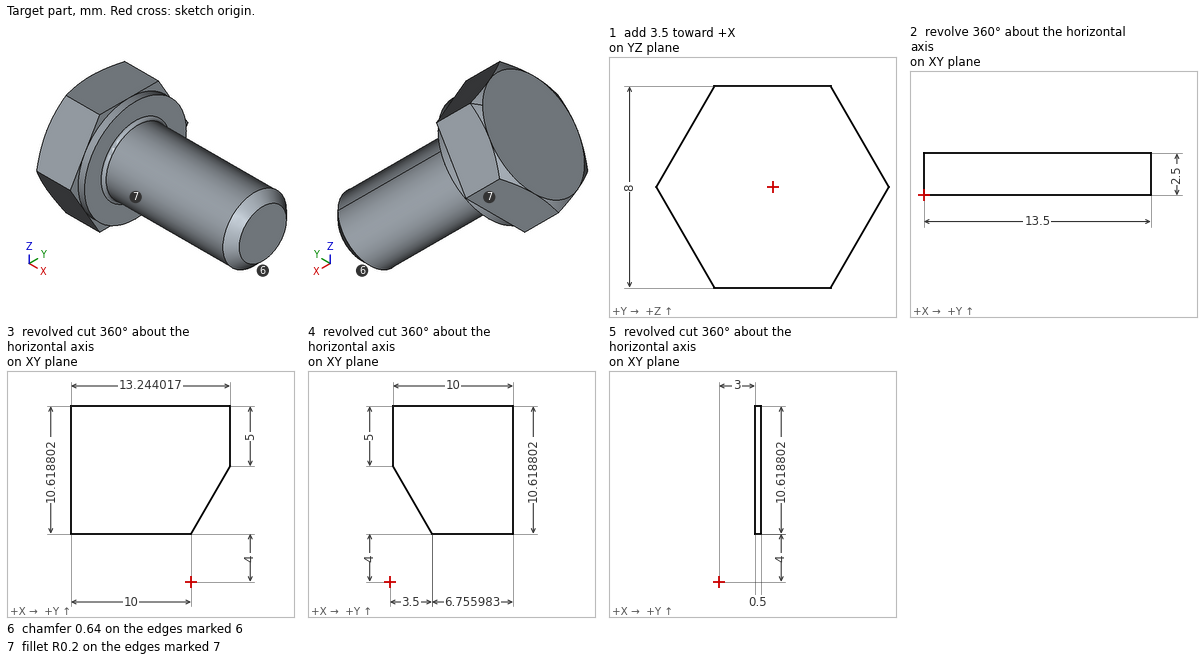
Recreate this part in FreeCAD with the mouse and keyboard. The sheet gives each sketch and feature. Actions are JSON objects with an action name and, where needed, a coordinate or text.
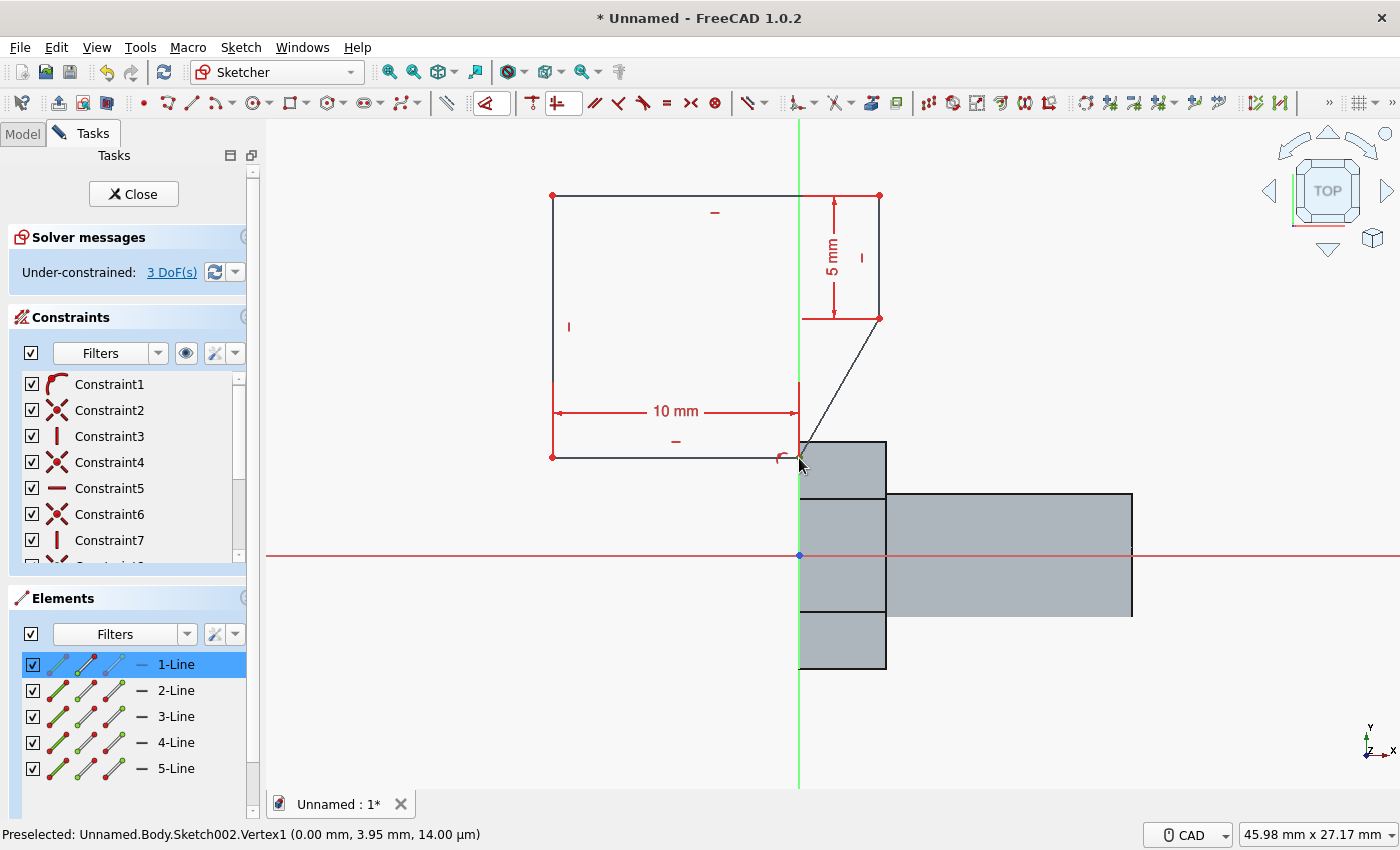
{"action": "key", "text": "i"}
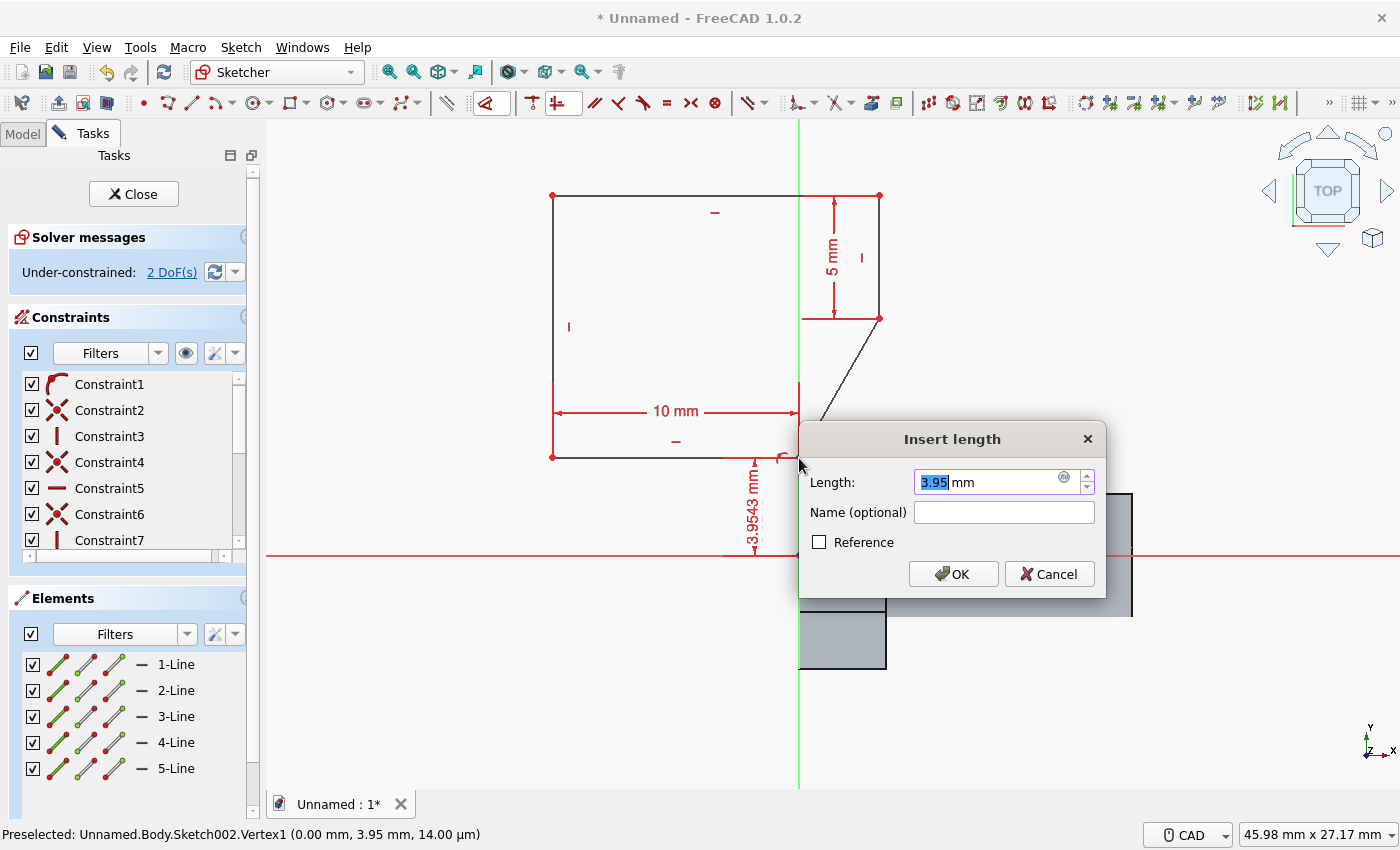
{"action": "type", "text": "4"}
{"action": "key", "text": "Return"}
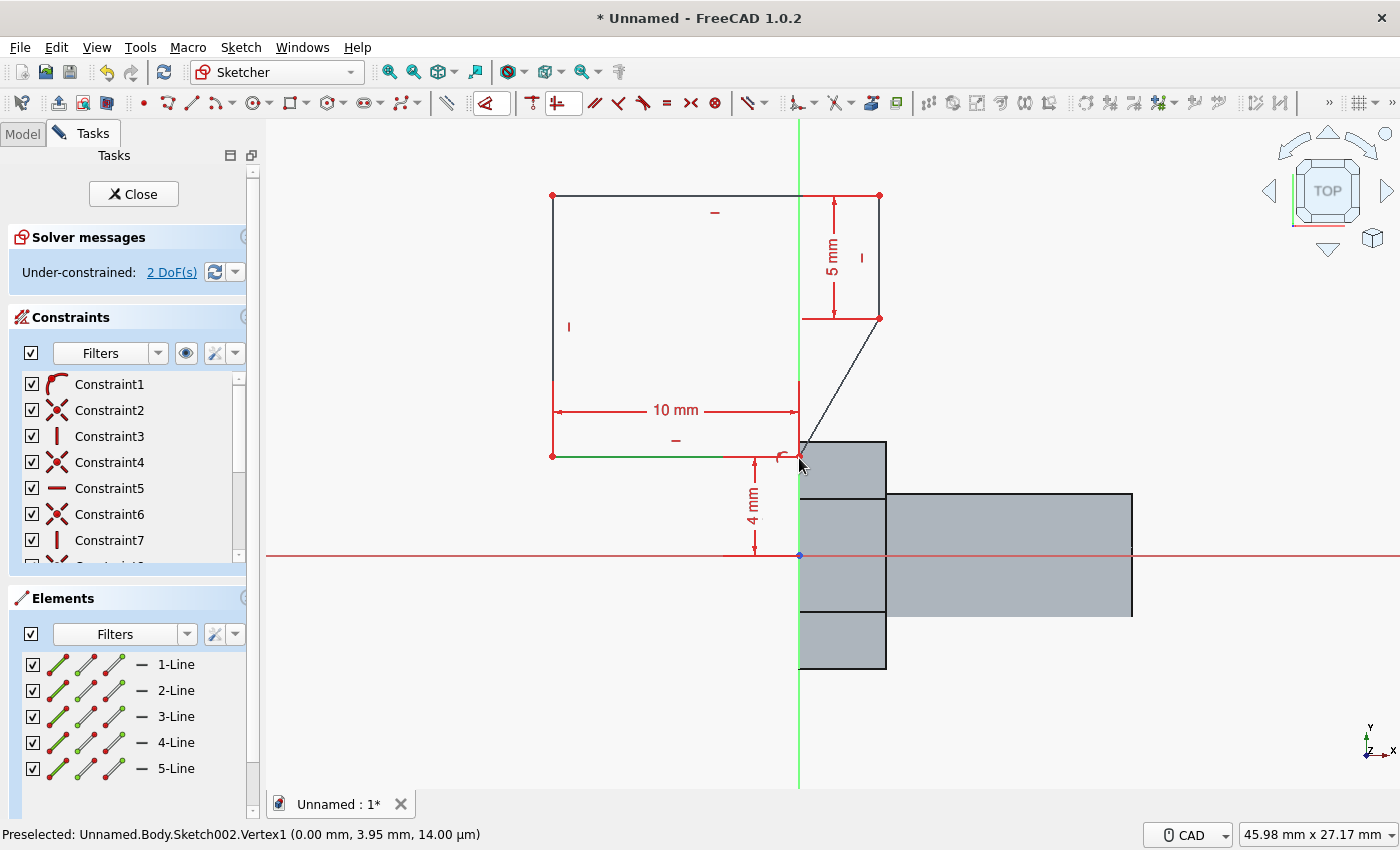
{"action": "left_click", "coordinate": [781, 196]}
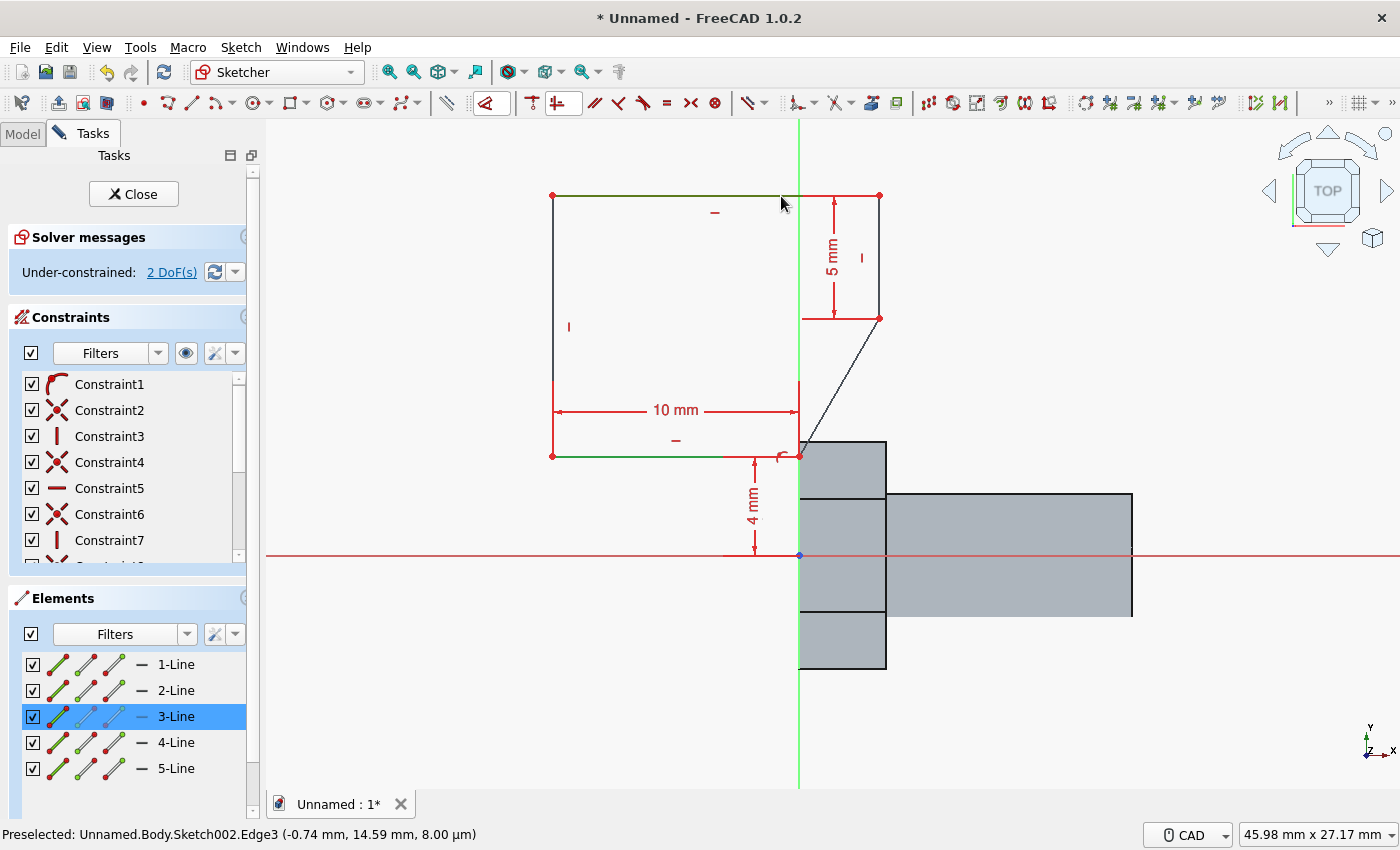
{"action": "left_click", "coordinate": [504, 104]}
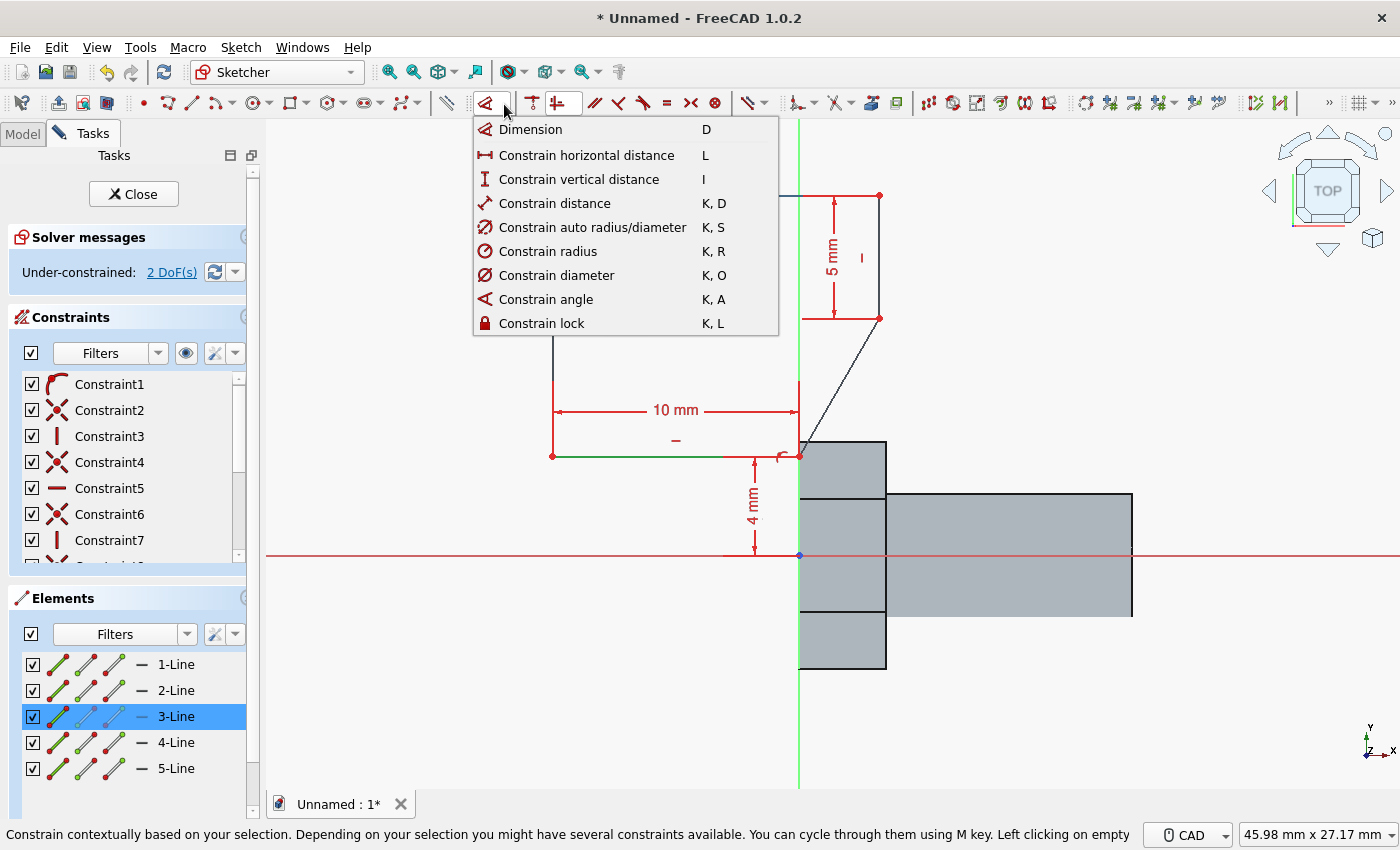
{"action": "left_click", "coordinate": [626, 155]}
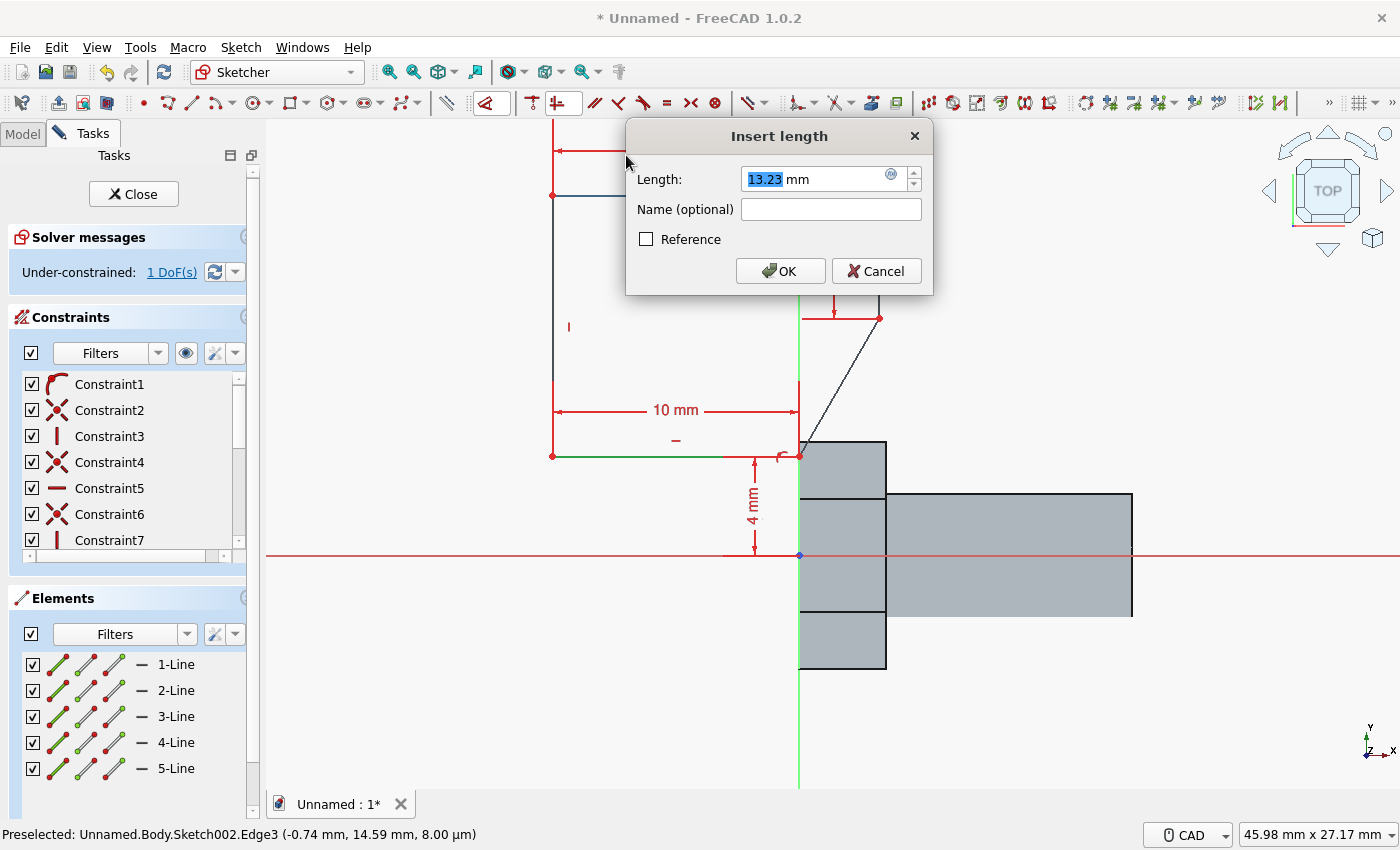
{"action": "type", "text": "13.244017"}
{"action": "key", "text": "Return"}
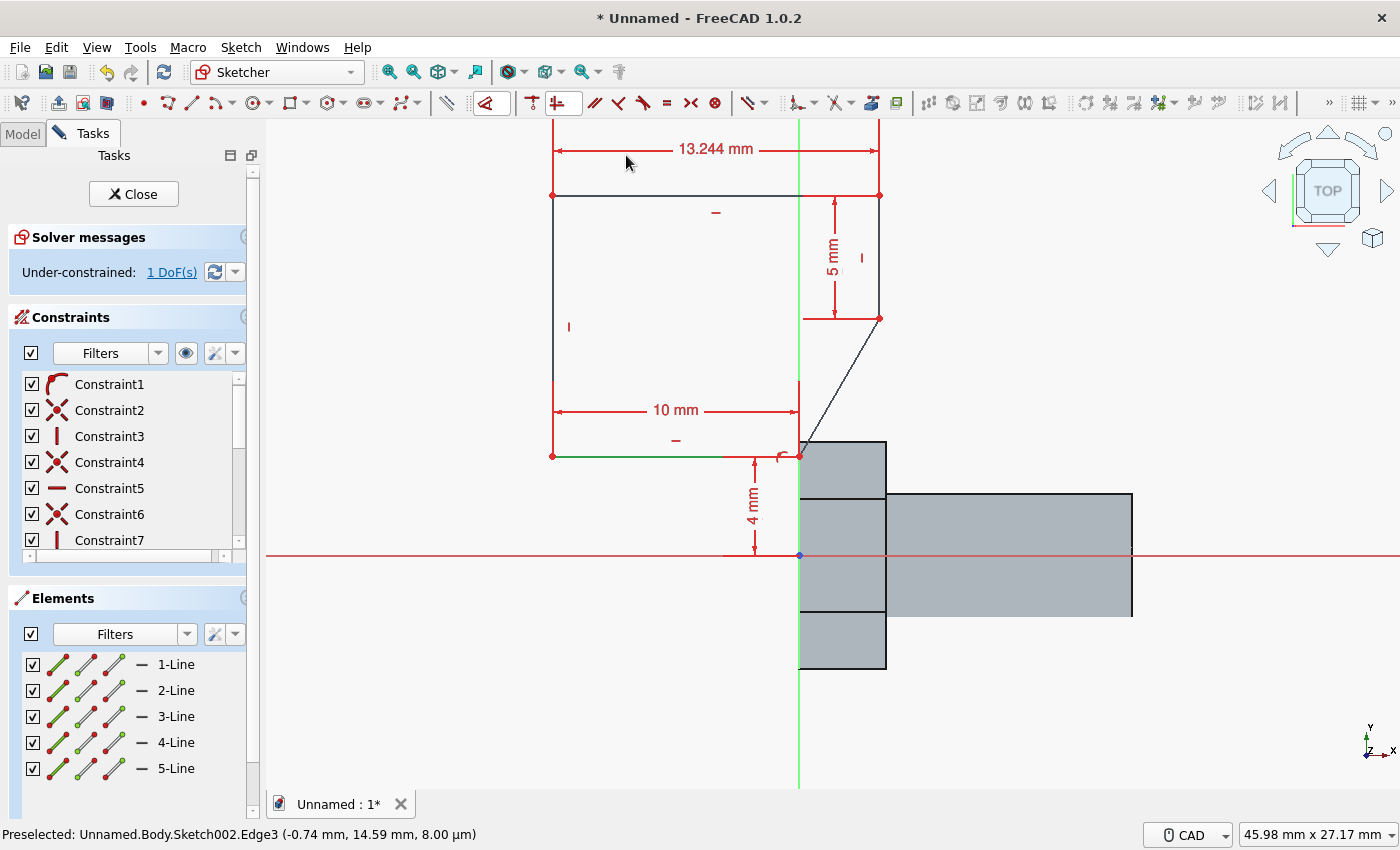
{"action": "left_click", "coordinate": [553, 274]}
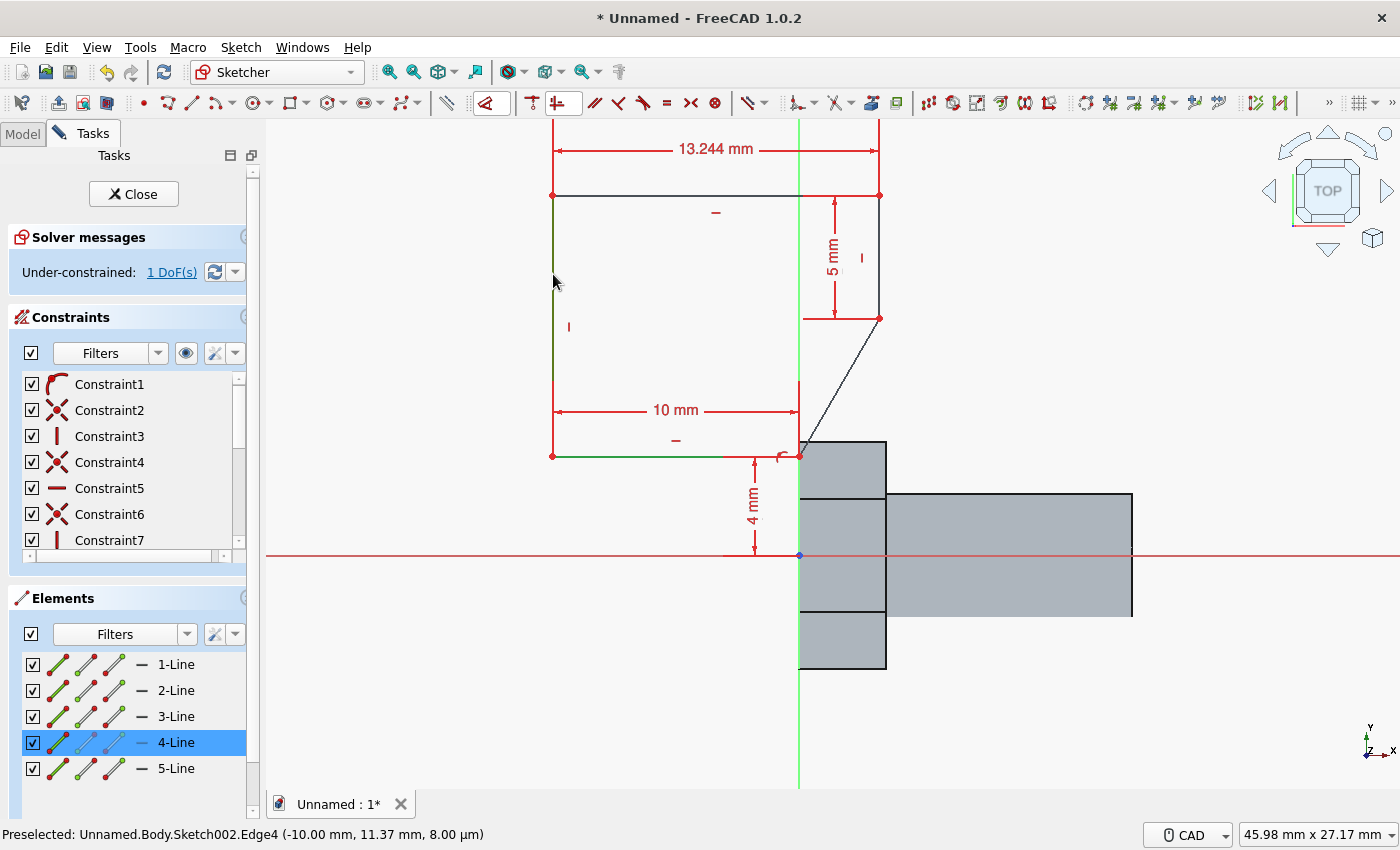
{"action": "key", "text": "i"}